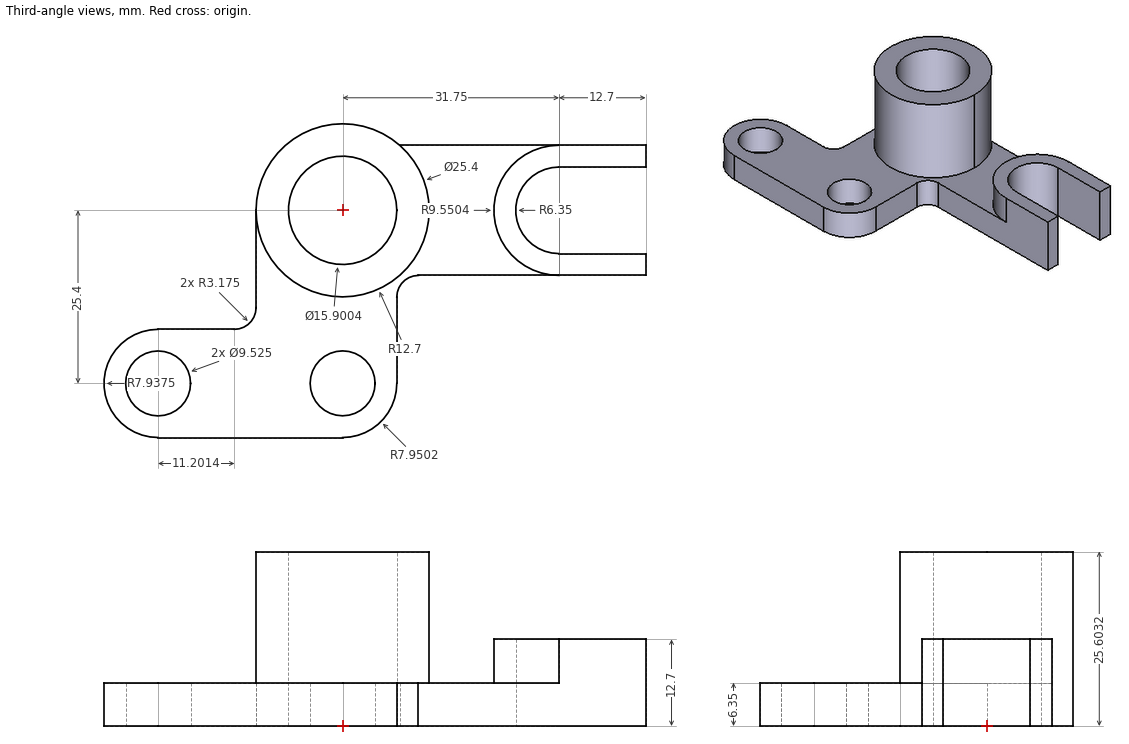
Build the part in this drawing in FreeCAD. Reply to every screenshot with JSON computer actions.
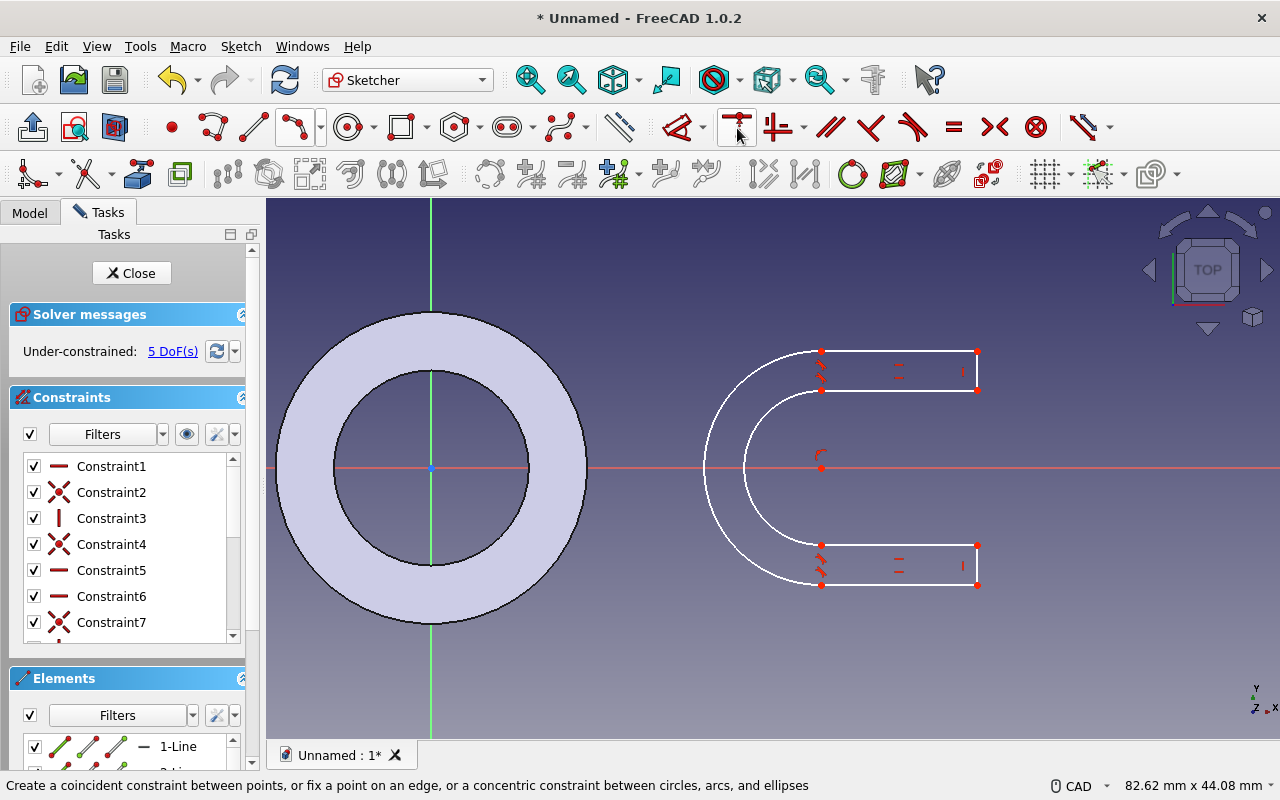
{"action": "left_click", "coordinate": [676, 128]}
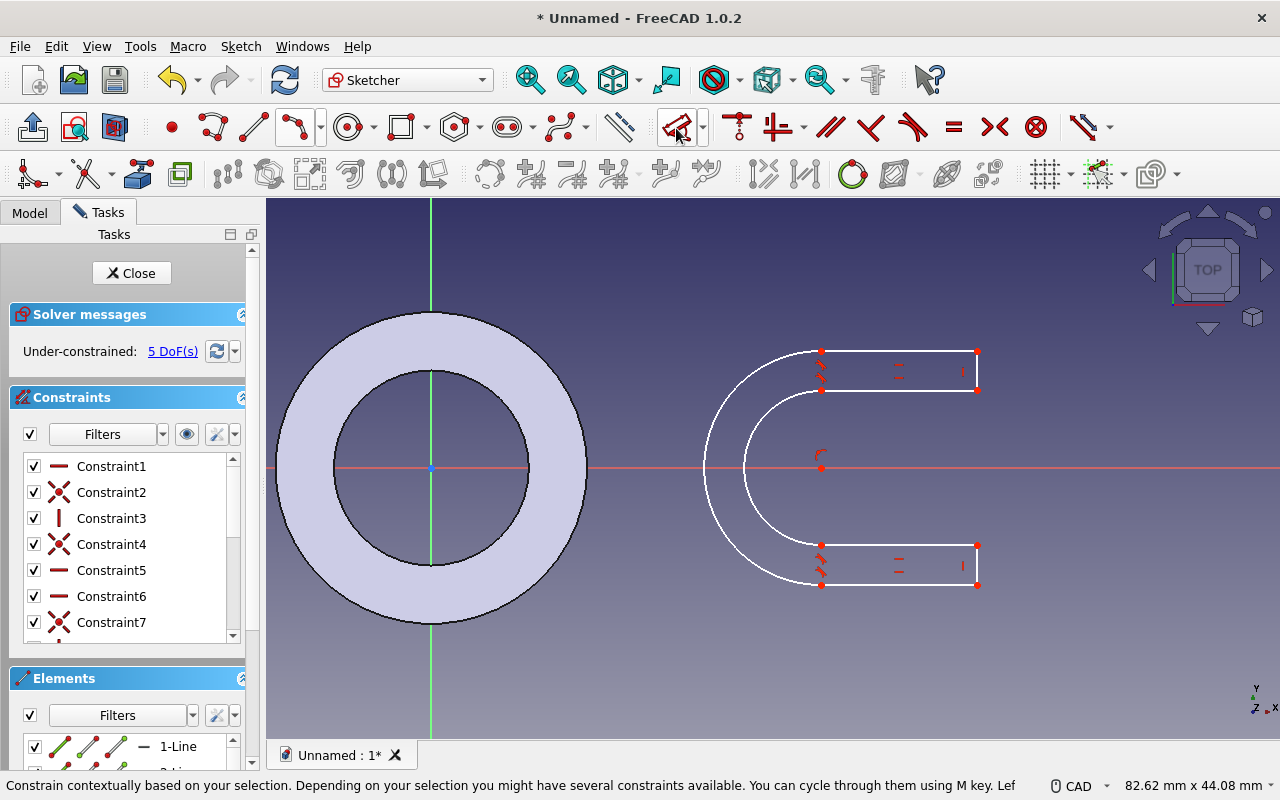
{"action": "left_click", "coordinate": [759, 423]}
{"action": "left_click", "coordinate": [909, 532]}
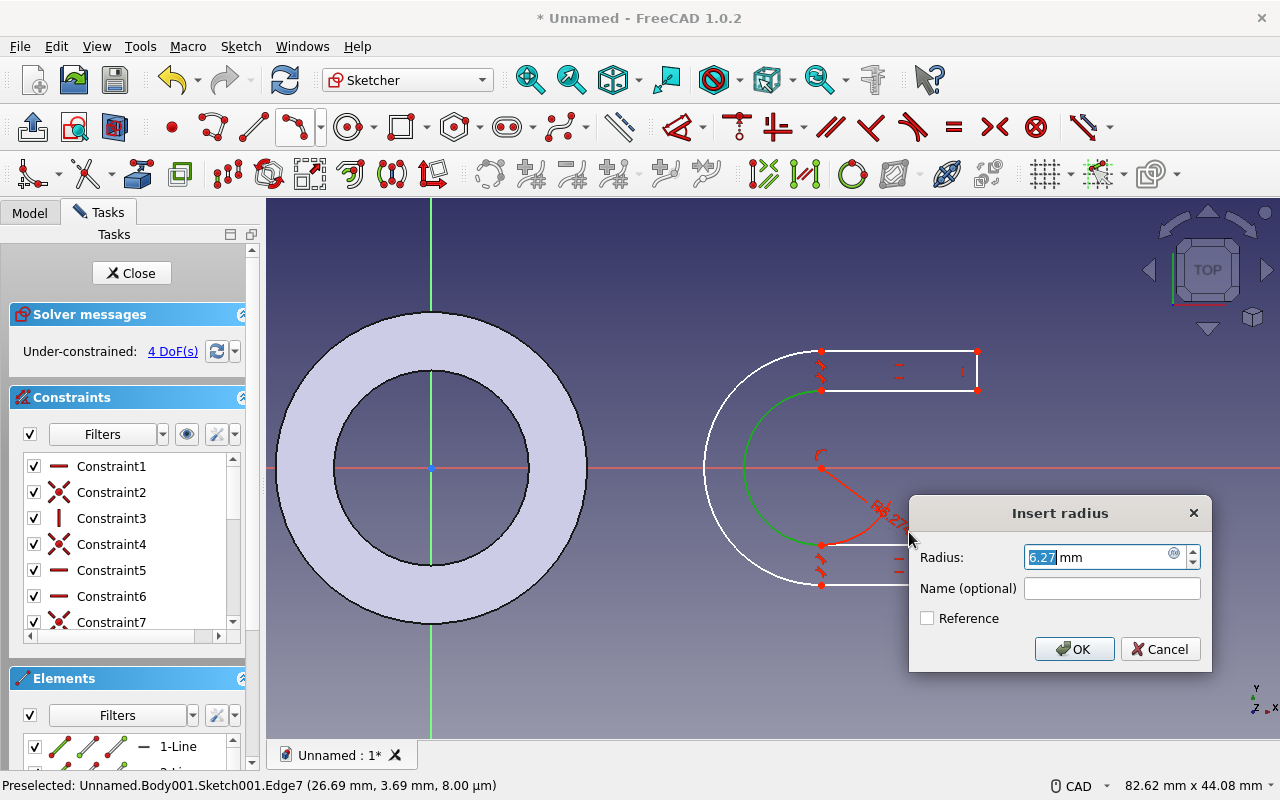
{"action": "type", "text": "6.35"}
{"action": "key", "text": "Return"}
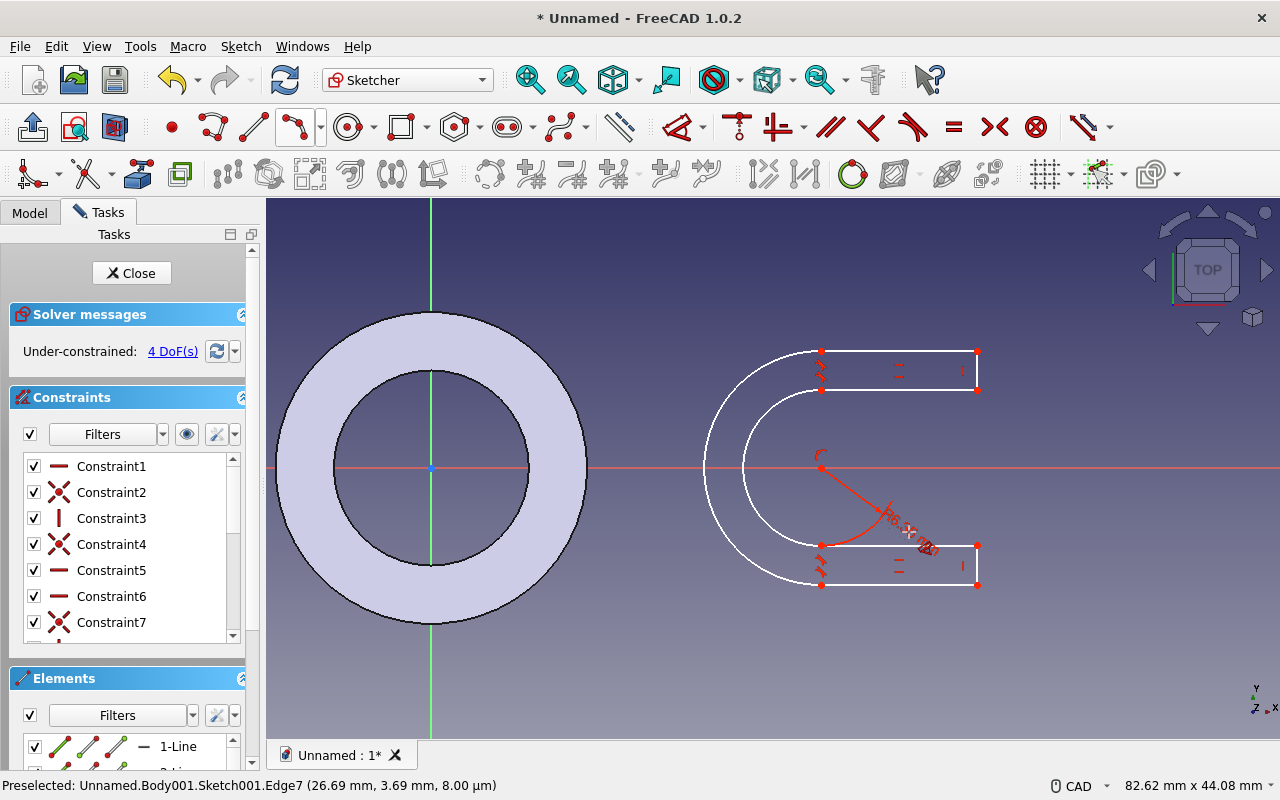
{"action": "left_click", "coordinate": [727, 399]}
{"action": "left_click", "coordinate": [701, 380]}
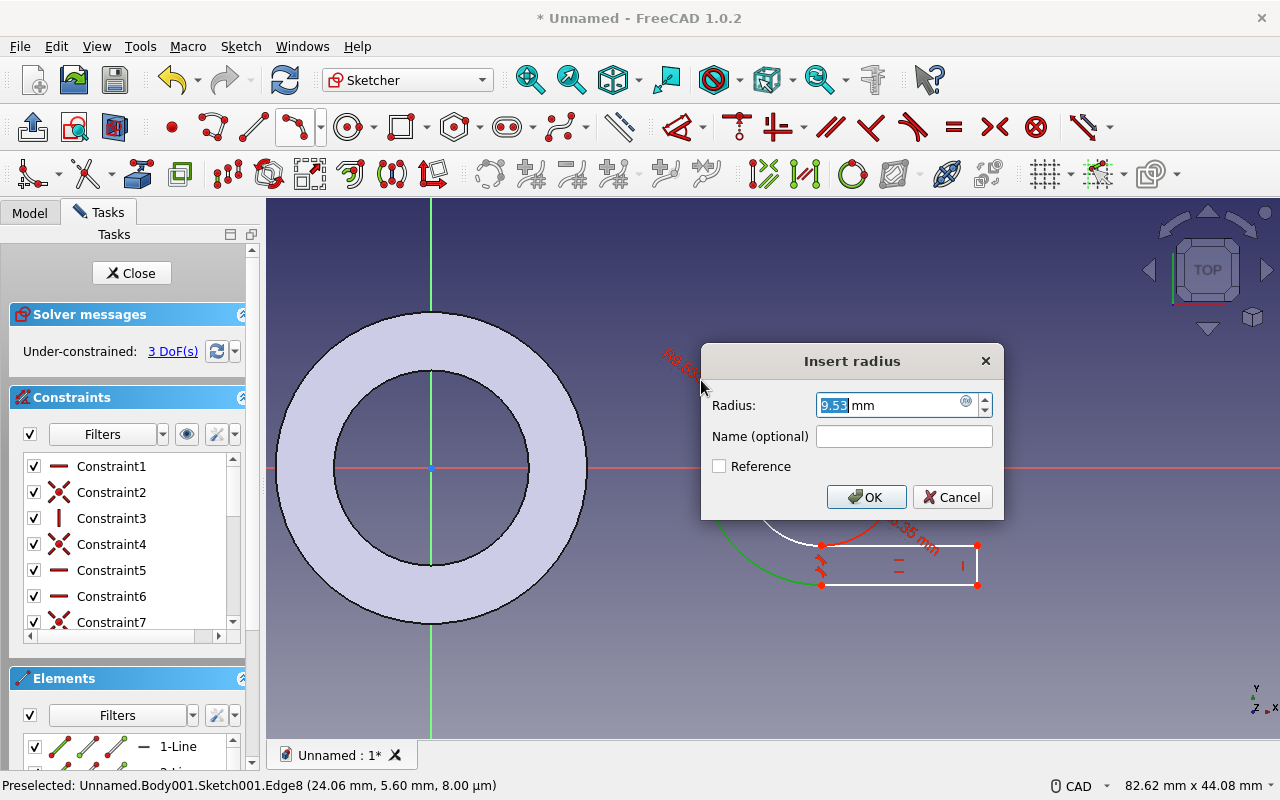
{"action": "type", "text": "9.5504"}
{"action": "key", "text": "Return"}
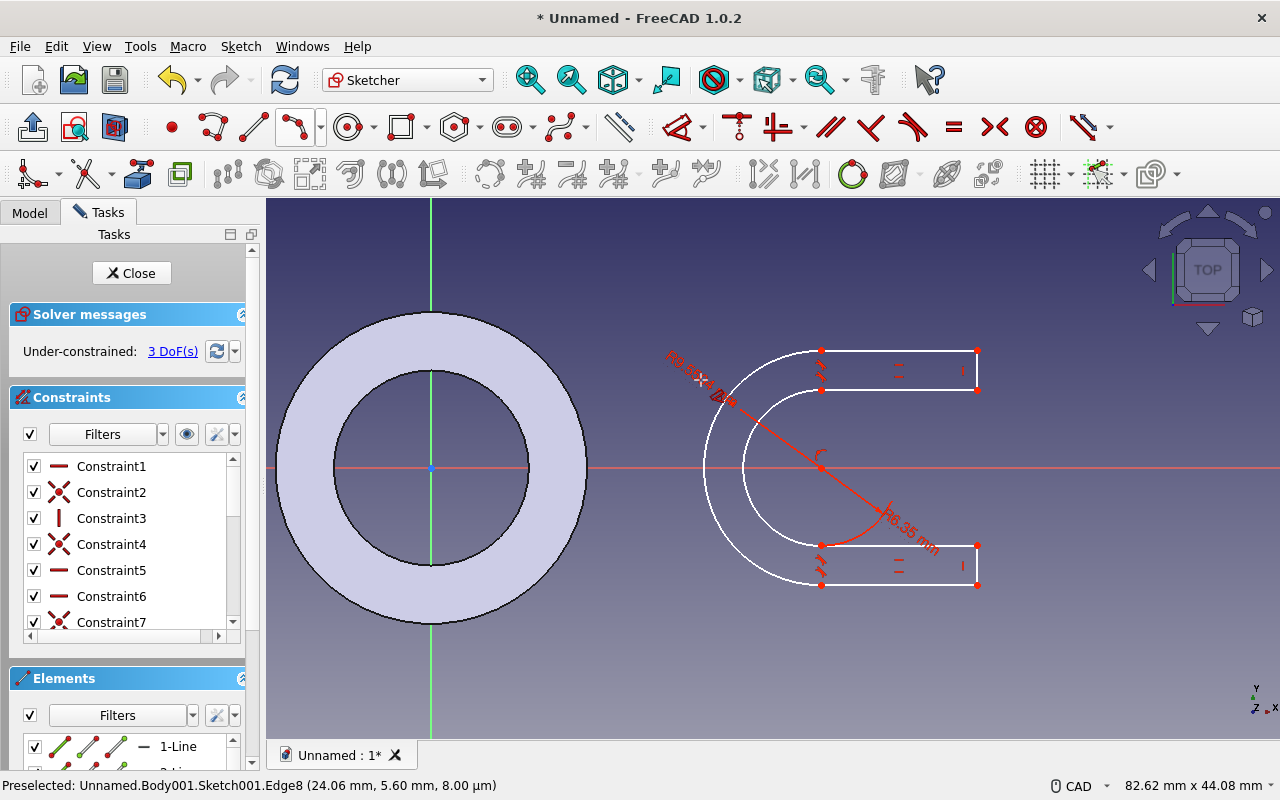
{"action": "left_click", "coordinate": [868, 585]}
{"action": "left_click", "coordinate": [899, 619]}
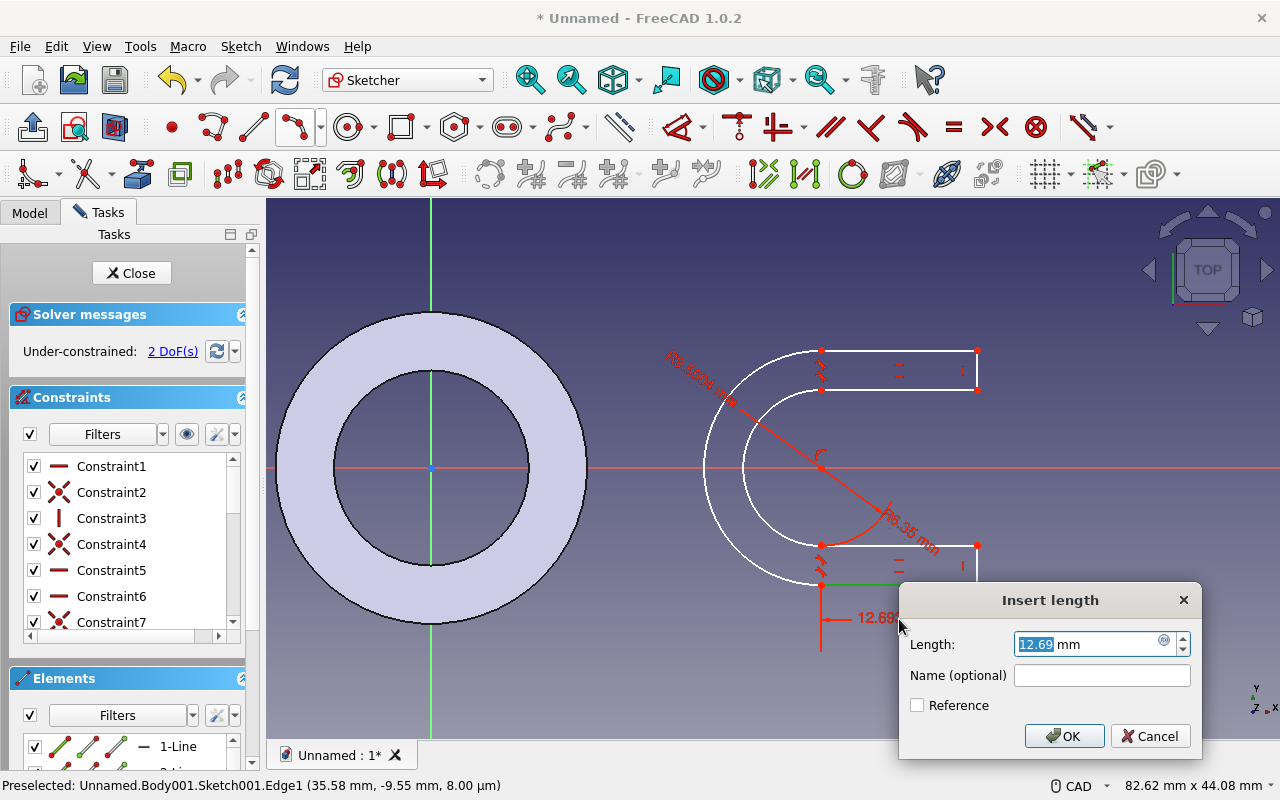
{"action": "type", "text": "12.7"}
{"action": "key", "text": "Return"}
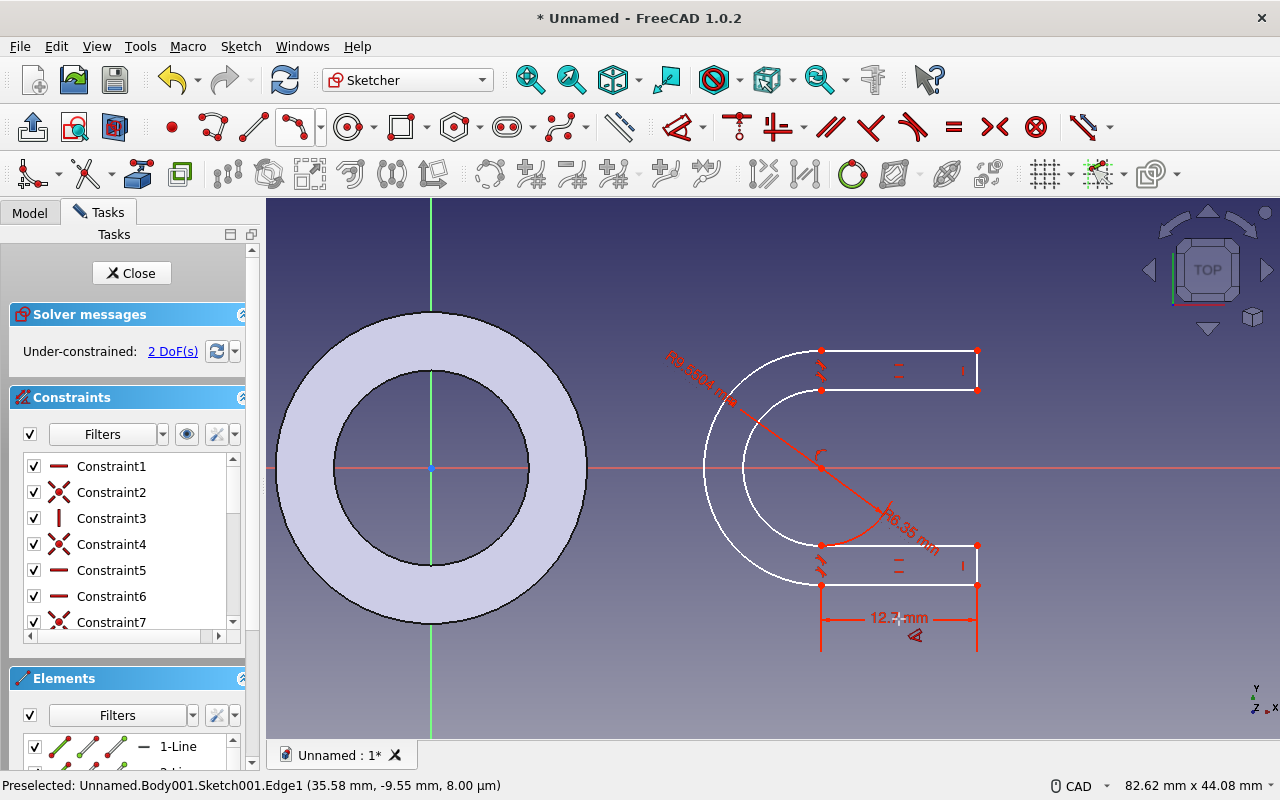
{"action": "left_click", "coordinate": [868, 390]}
{"action": "left_click", "coordinate": [899, 424]}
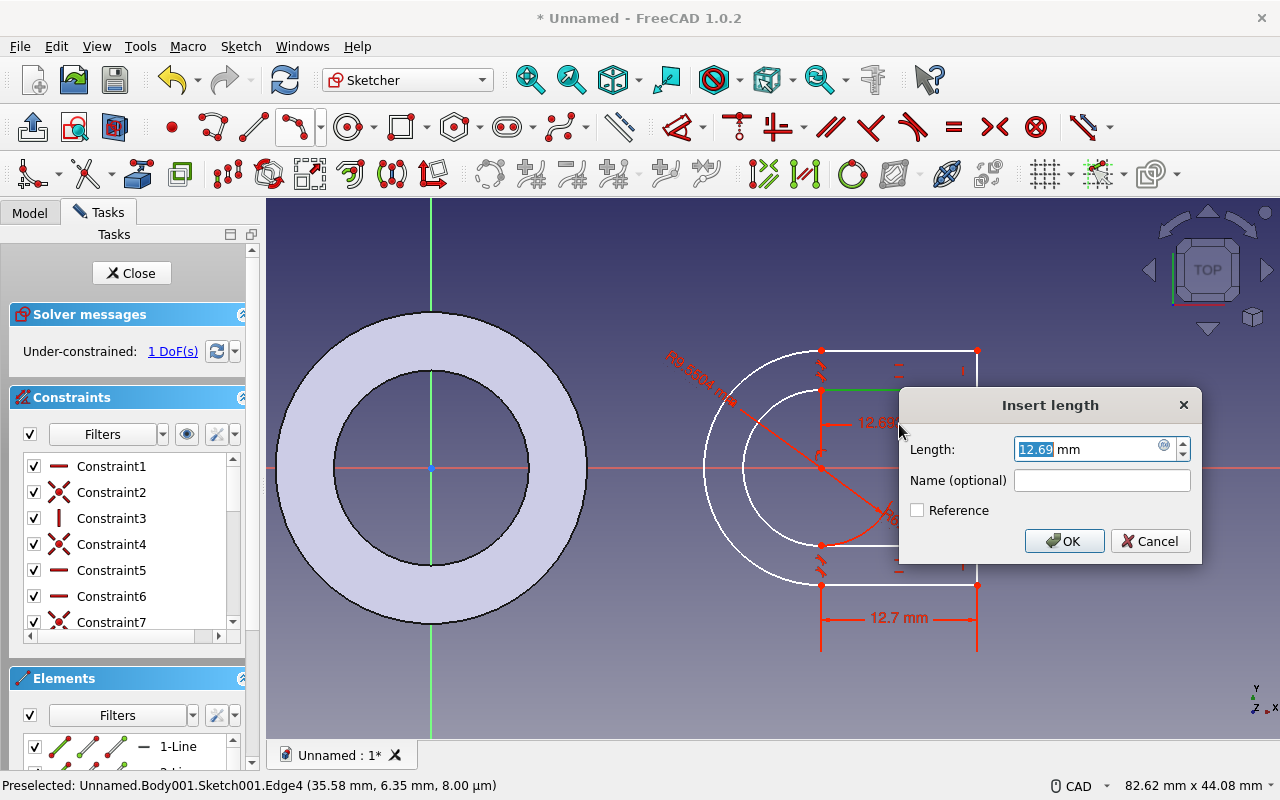
{"action": "type", "text": "12.7"}
{"action": "key", "text": "Return"}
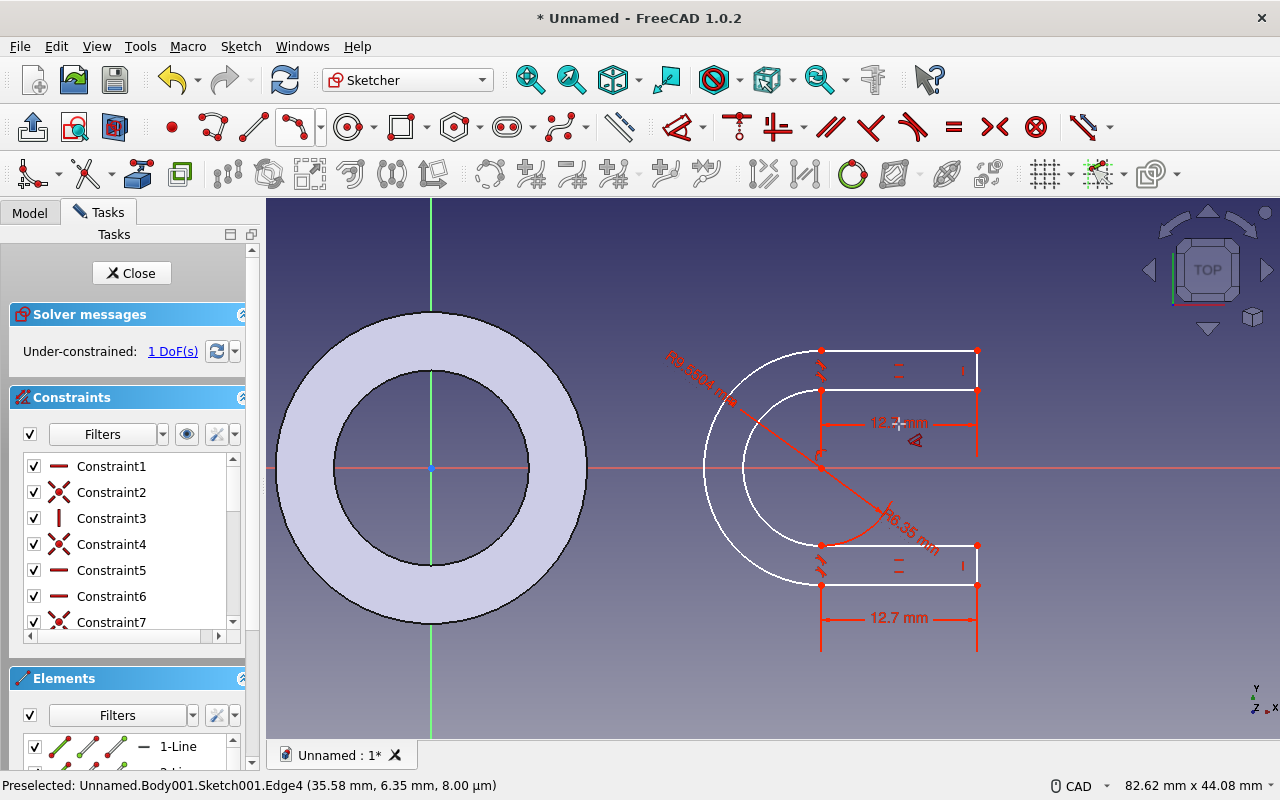
{"action": "left_click", "coordinate": [821, 585]}
{"action": "left_click", "coordinate": [626, 619]}